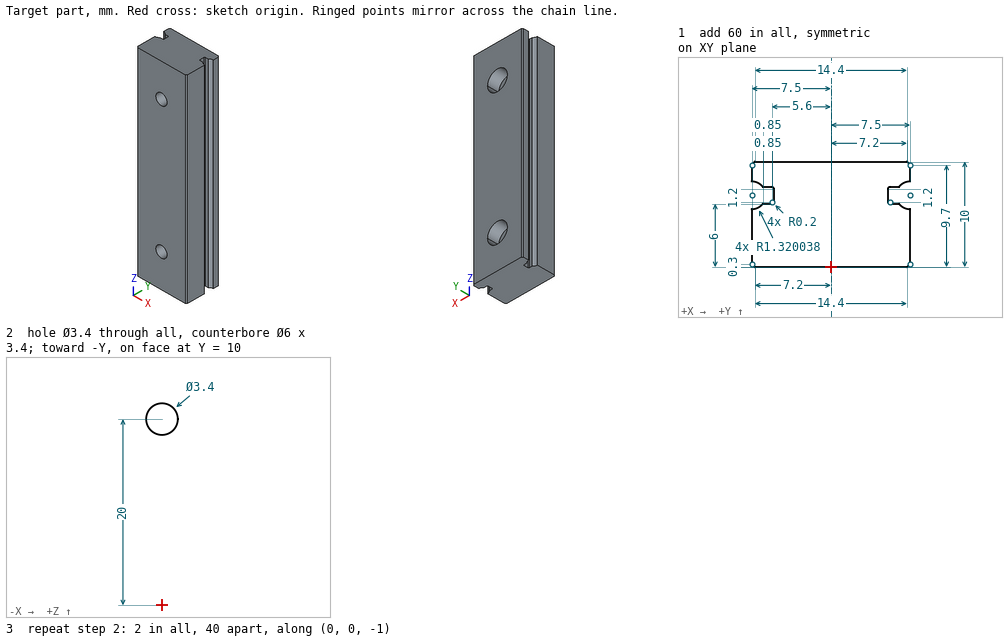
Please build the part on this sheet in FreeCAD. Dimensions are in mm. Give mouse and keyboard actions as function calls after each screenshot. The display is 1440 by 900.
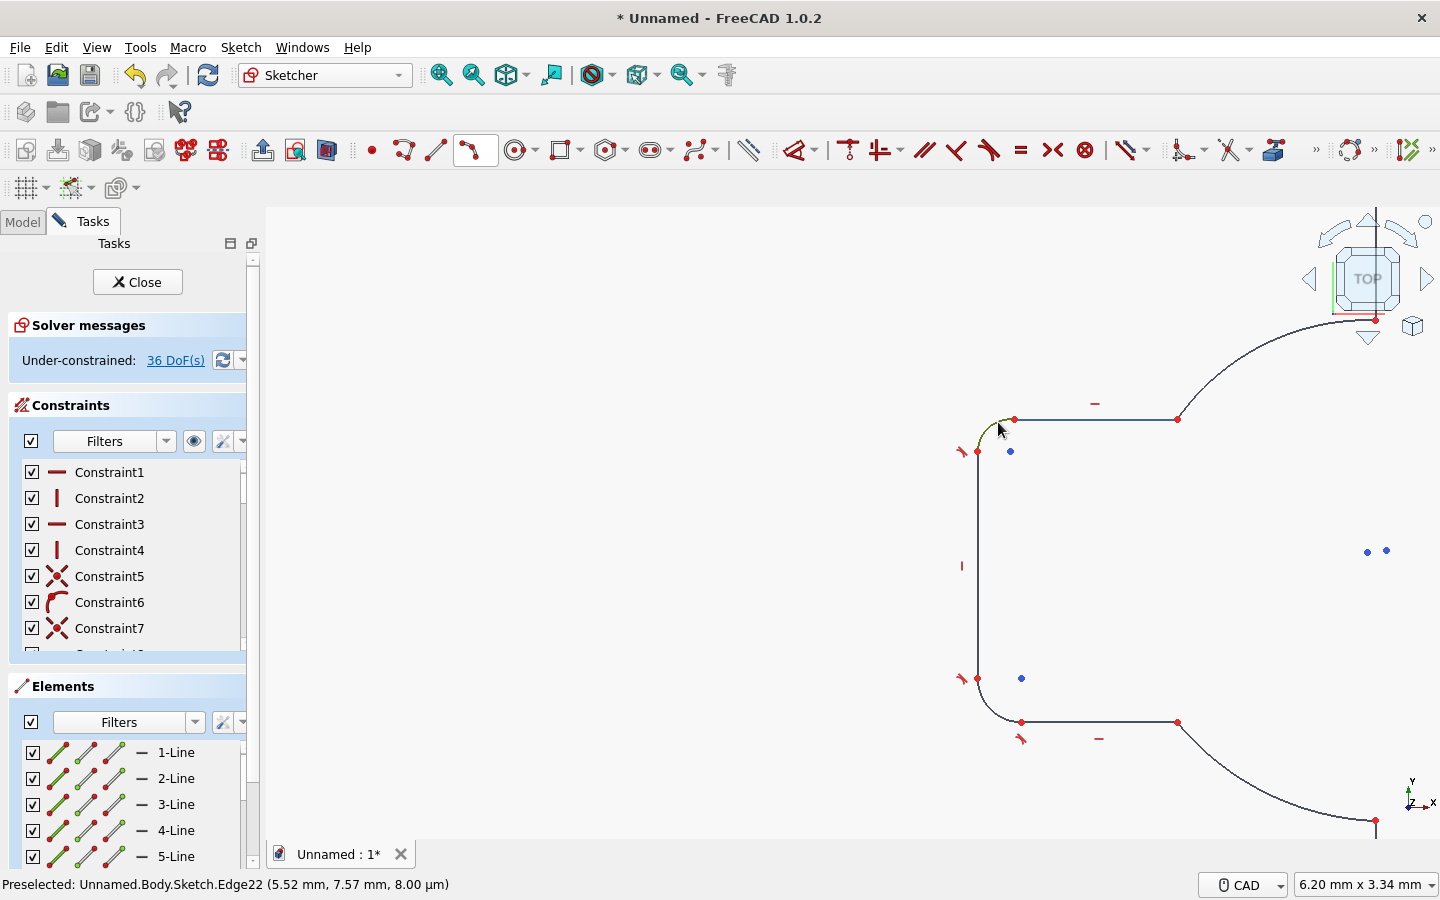
key(t)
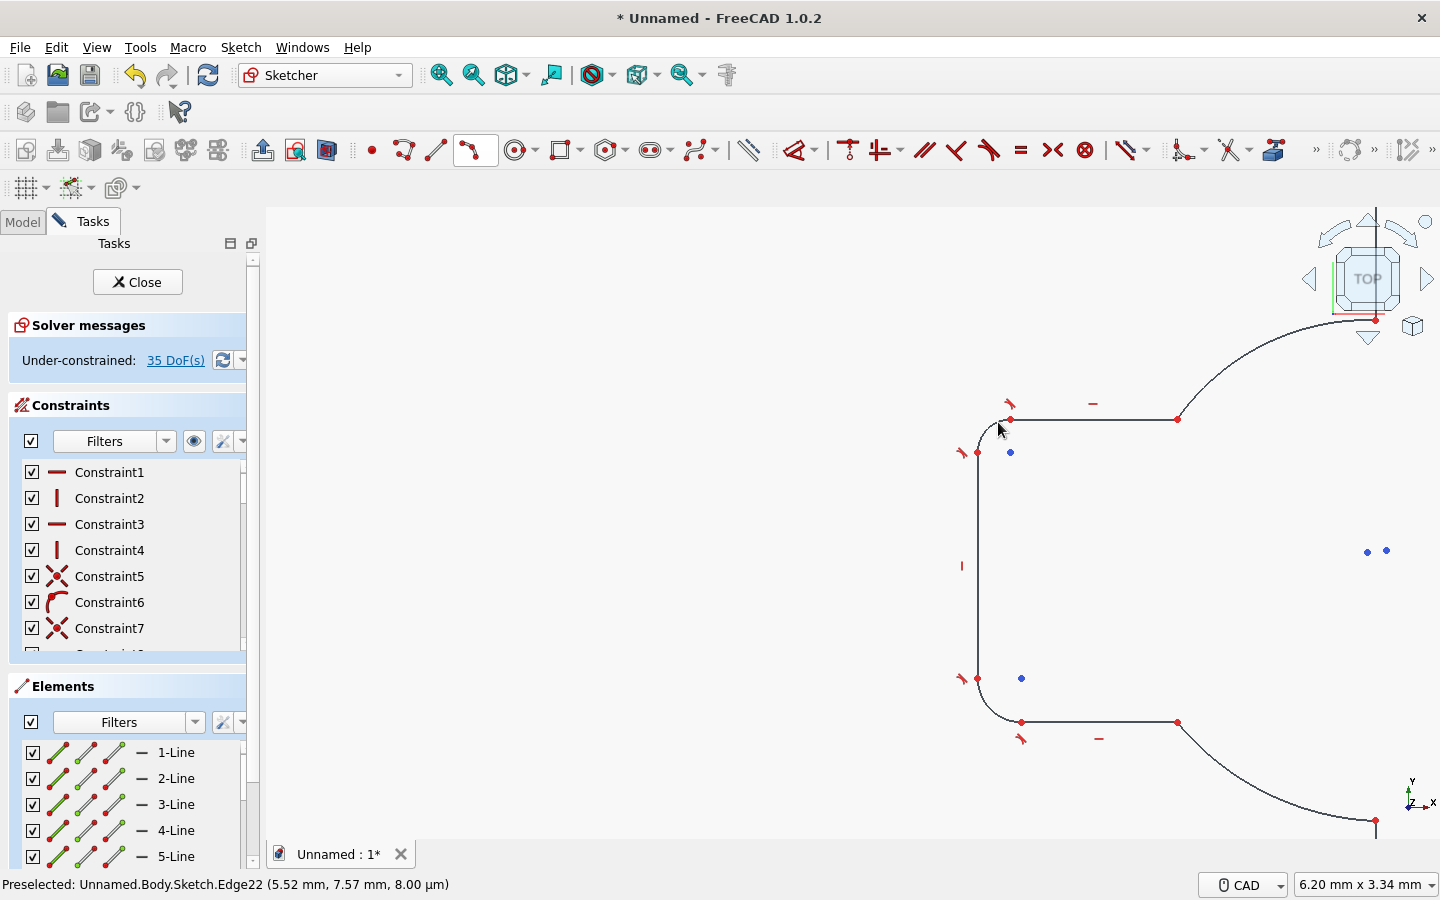
scroll(994, 426, down, 8)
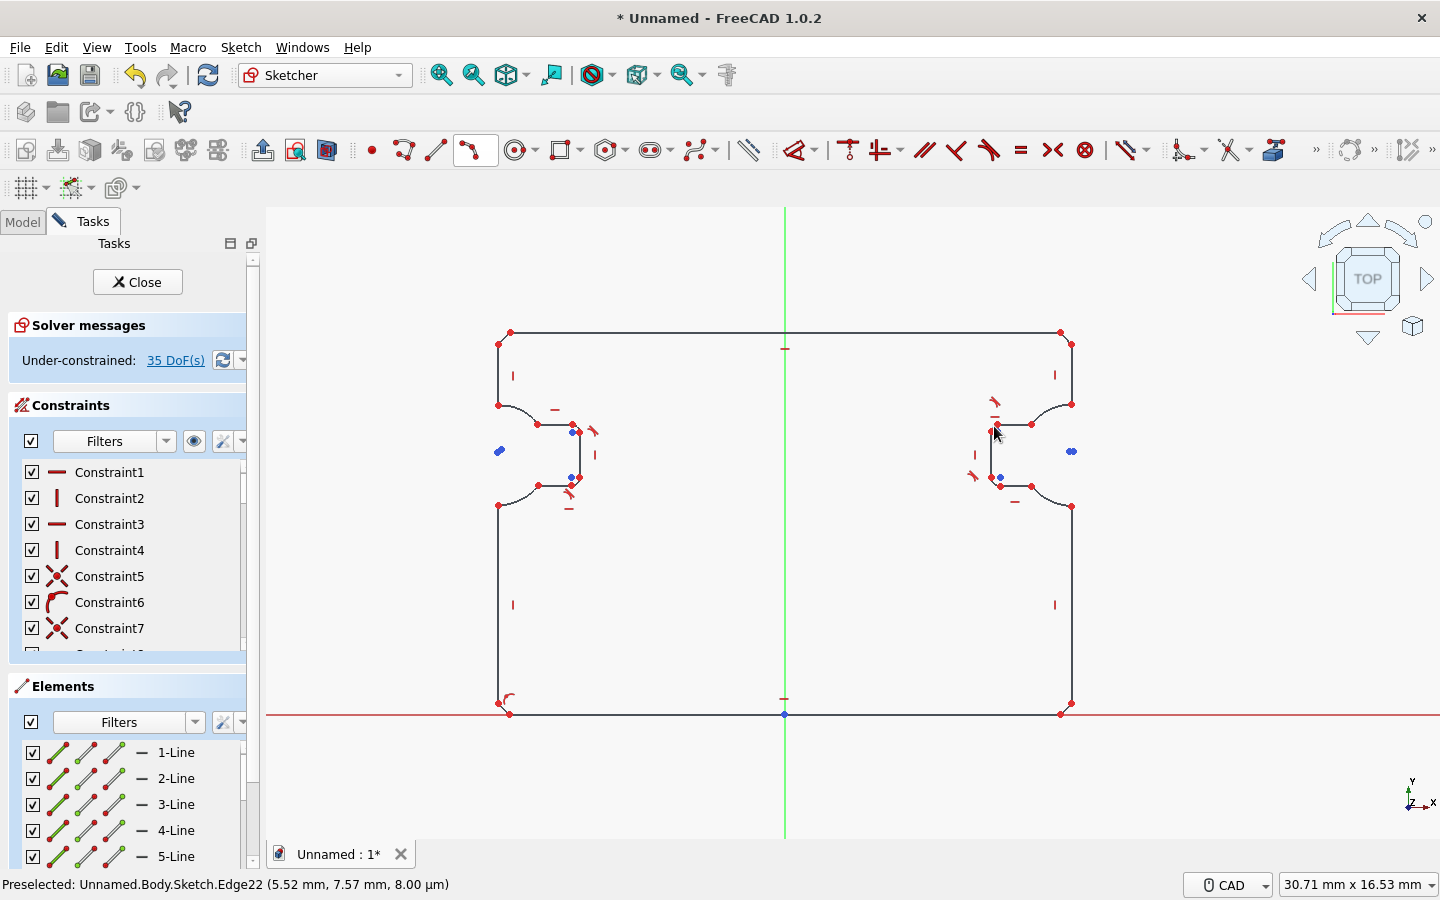
click(1041, 496)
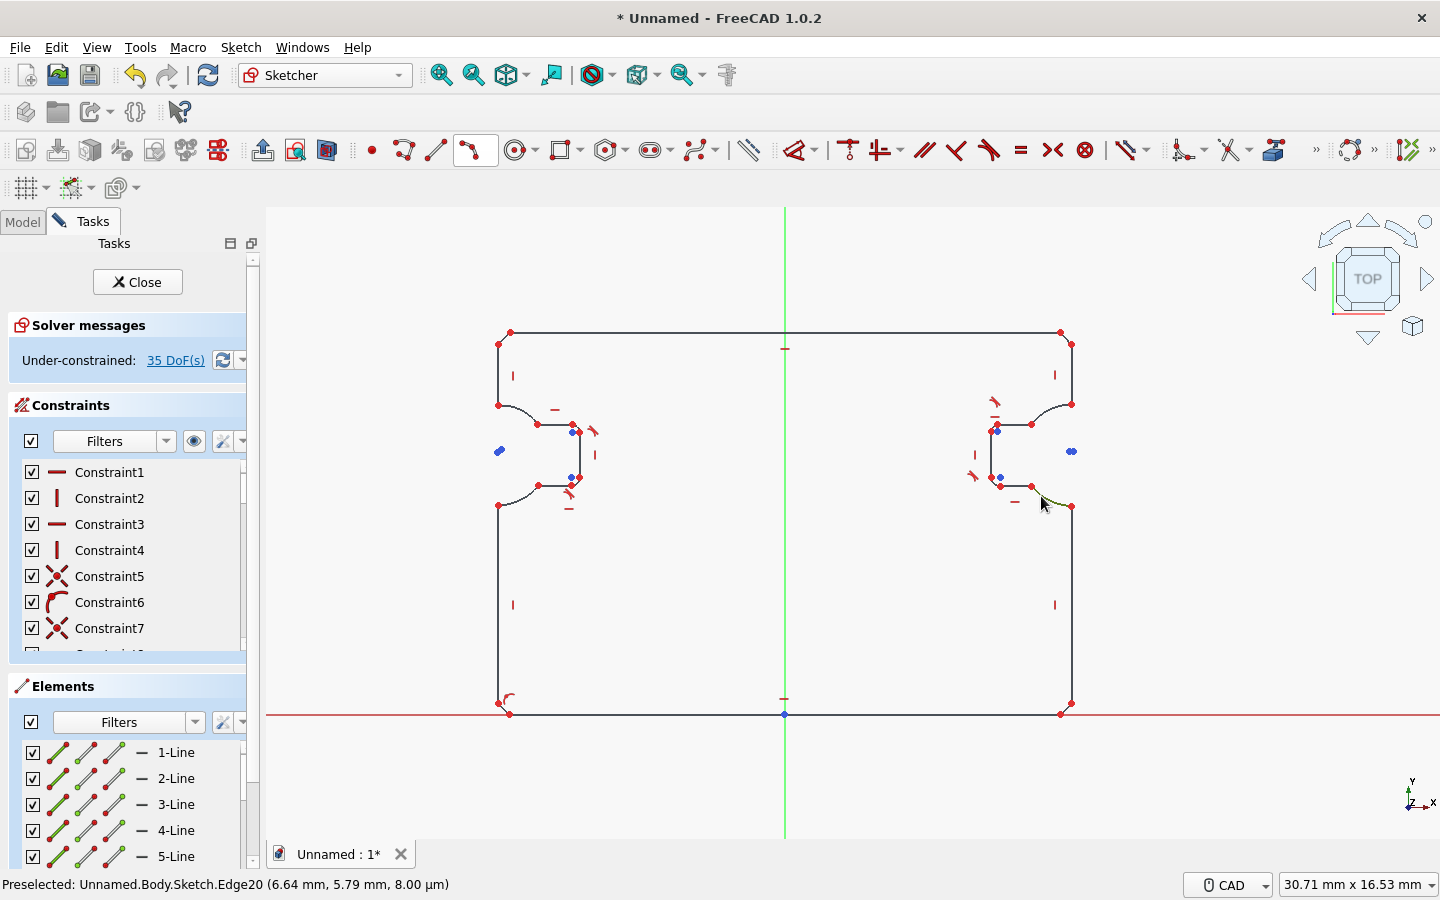
click(1058, 407)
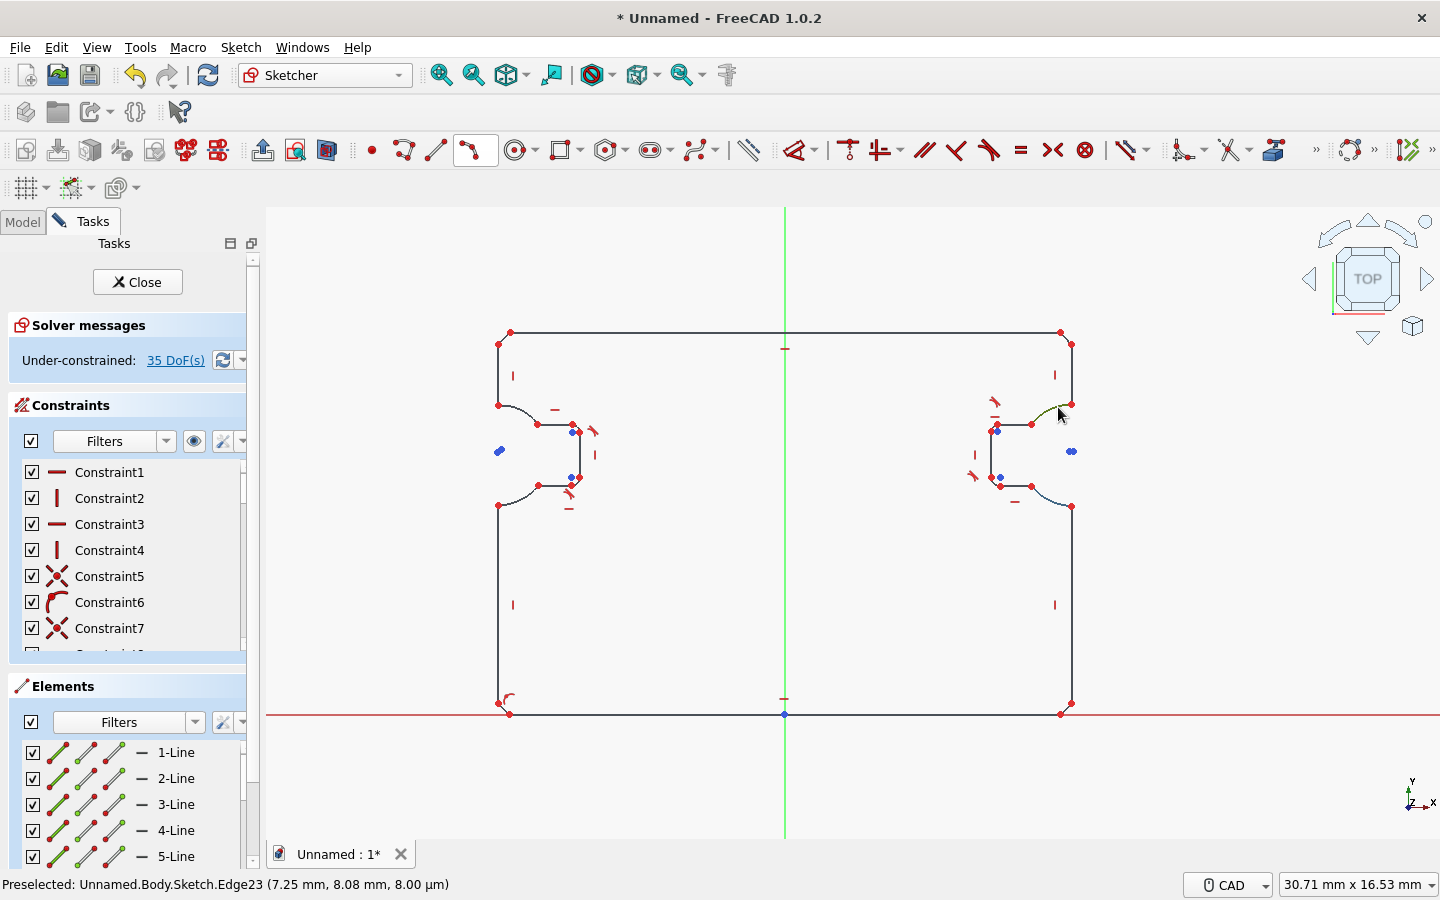
key(c)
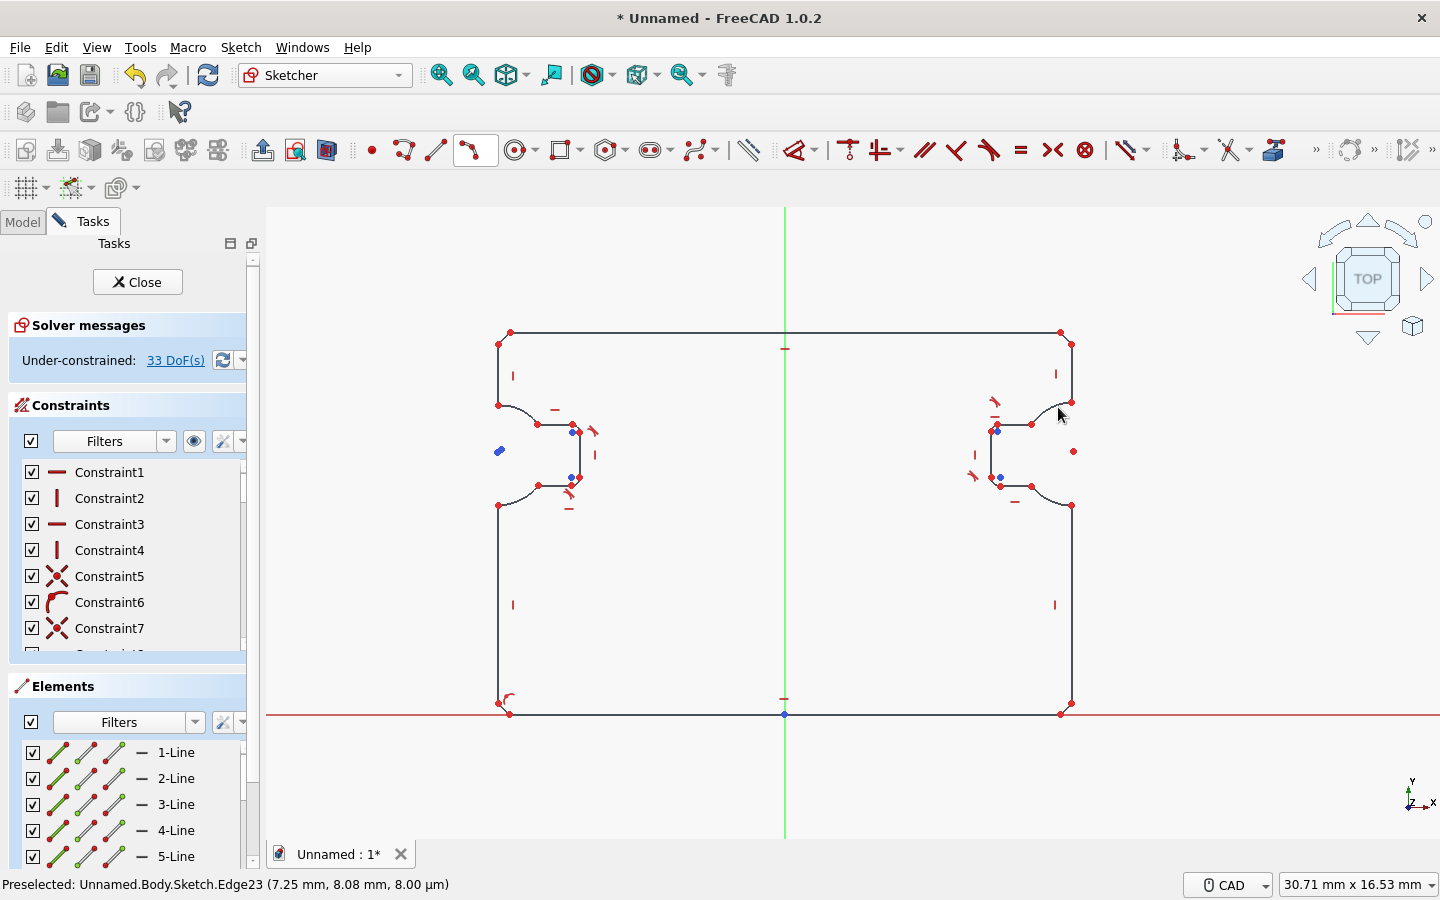
click(512, 503)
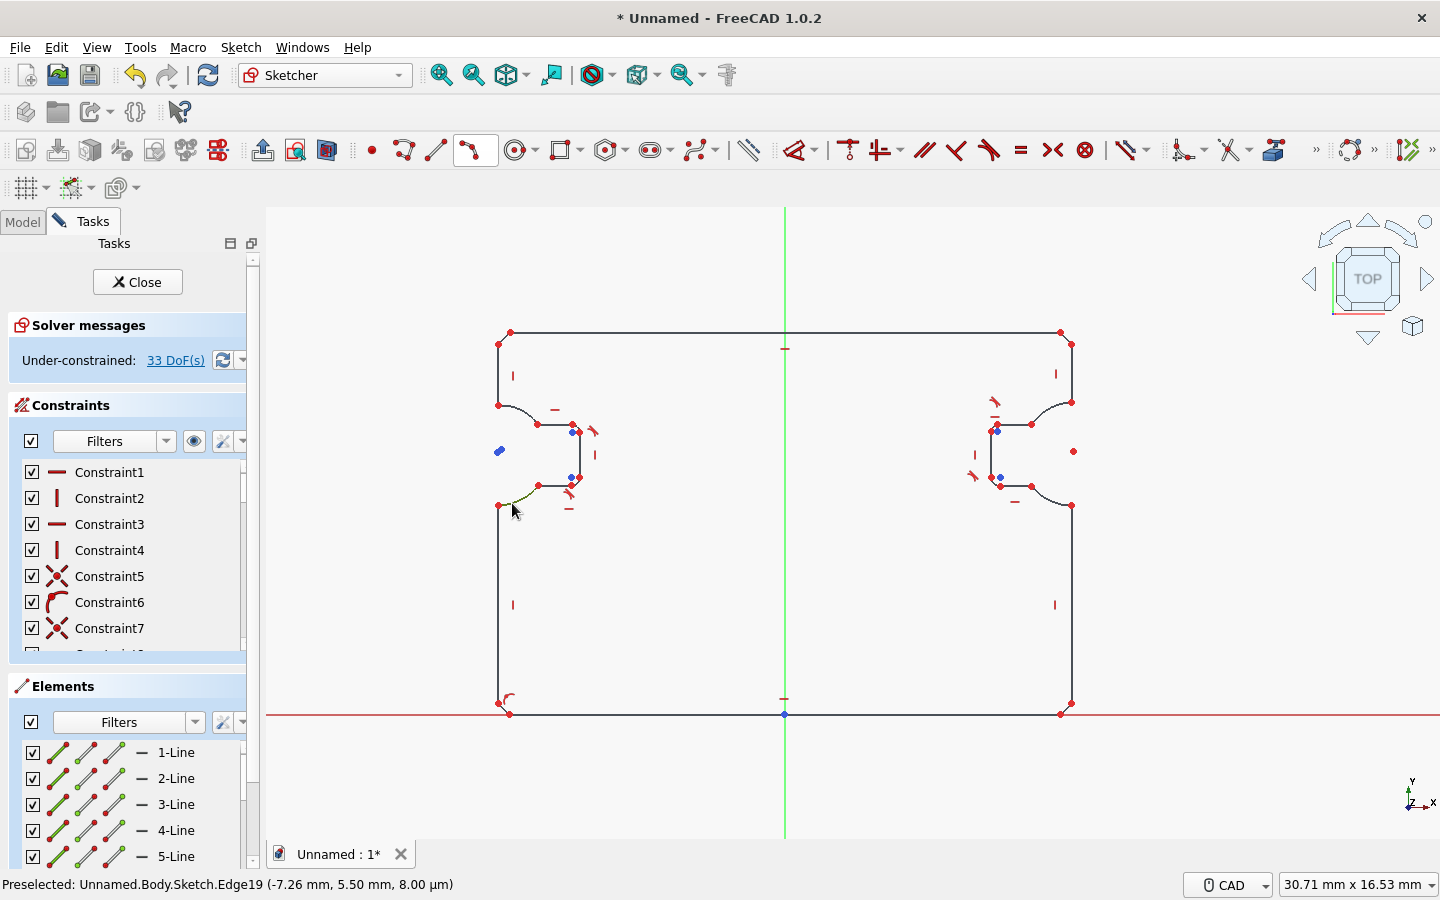
click(529, 415)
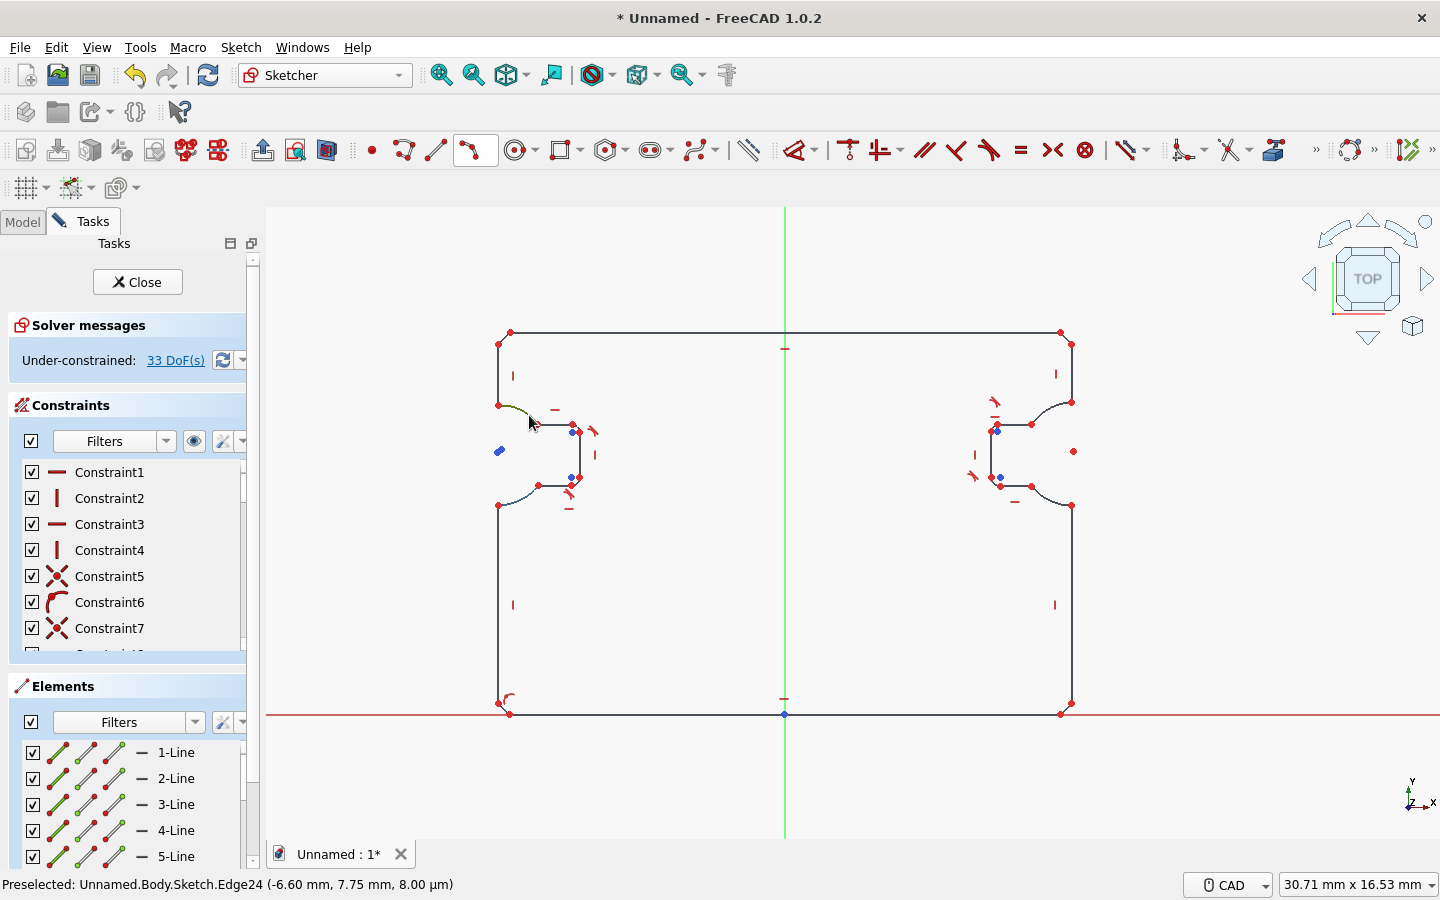
click(848, 150)